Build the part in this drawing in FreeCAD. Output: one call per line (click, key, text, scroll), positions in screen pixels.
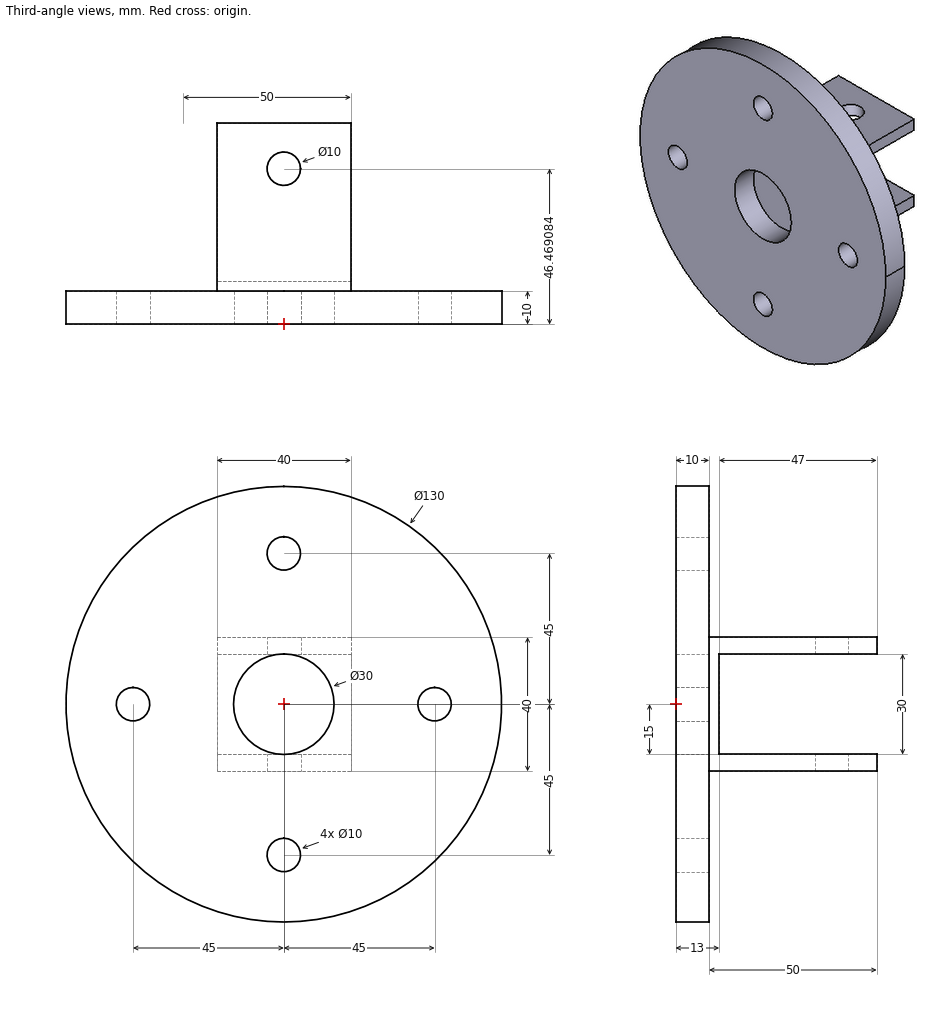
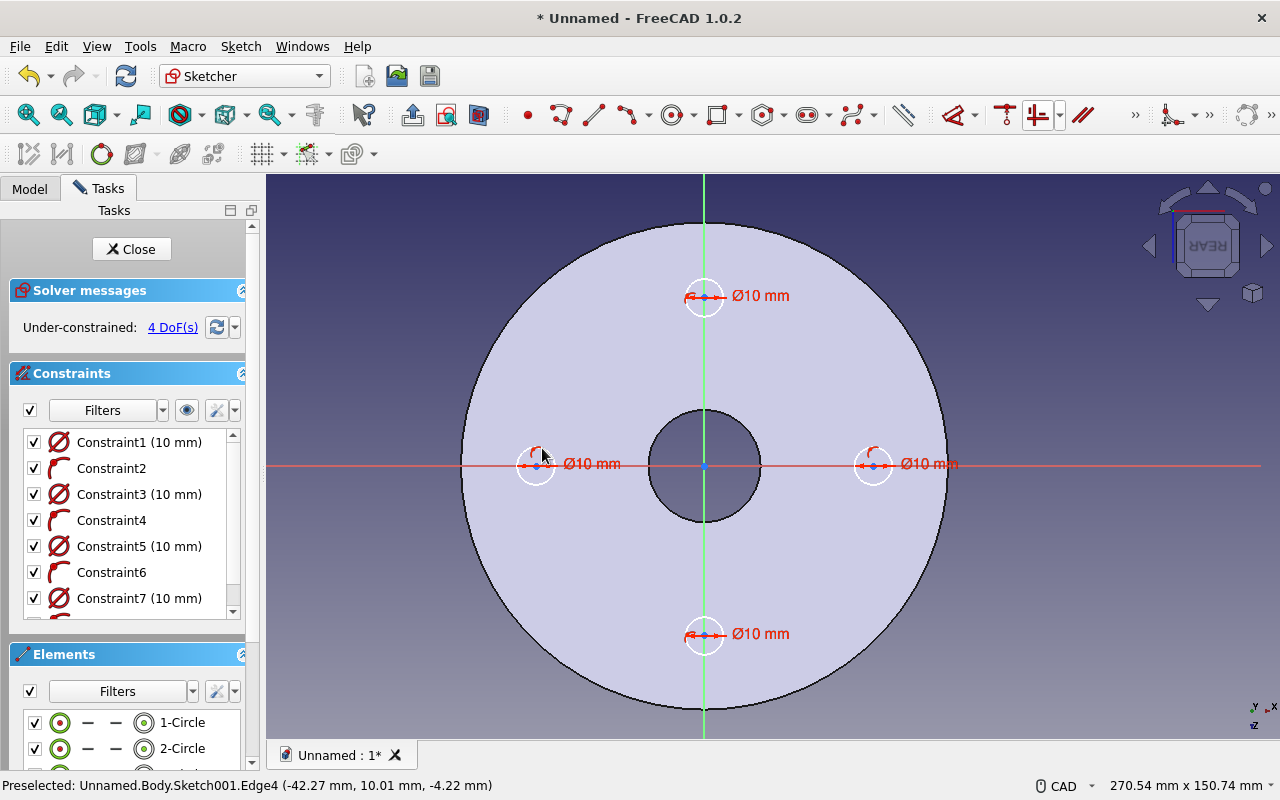
click(952, 116)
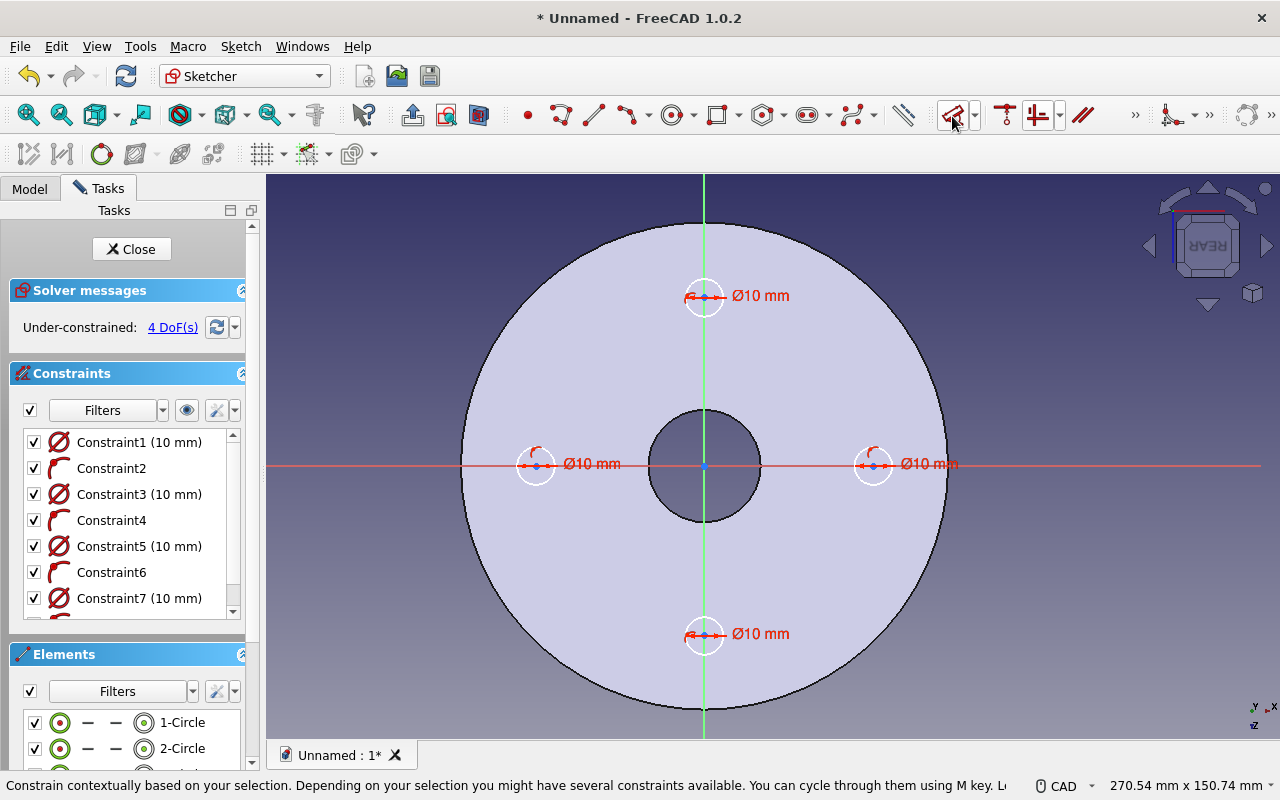
click(704, 298)
click(738, 382)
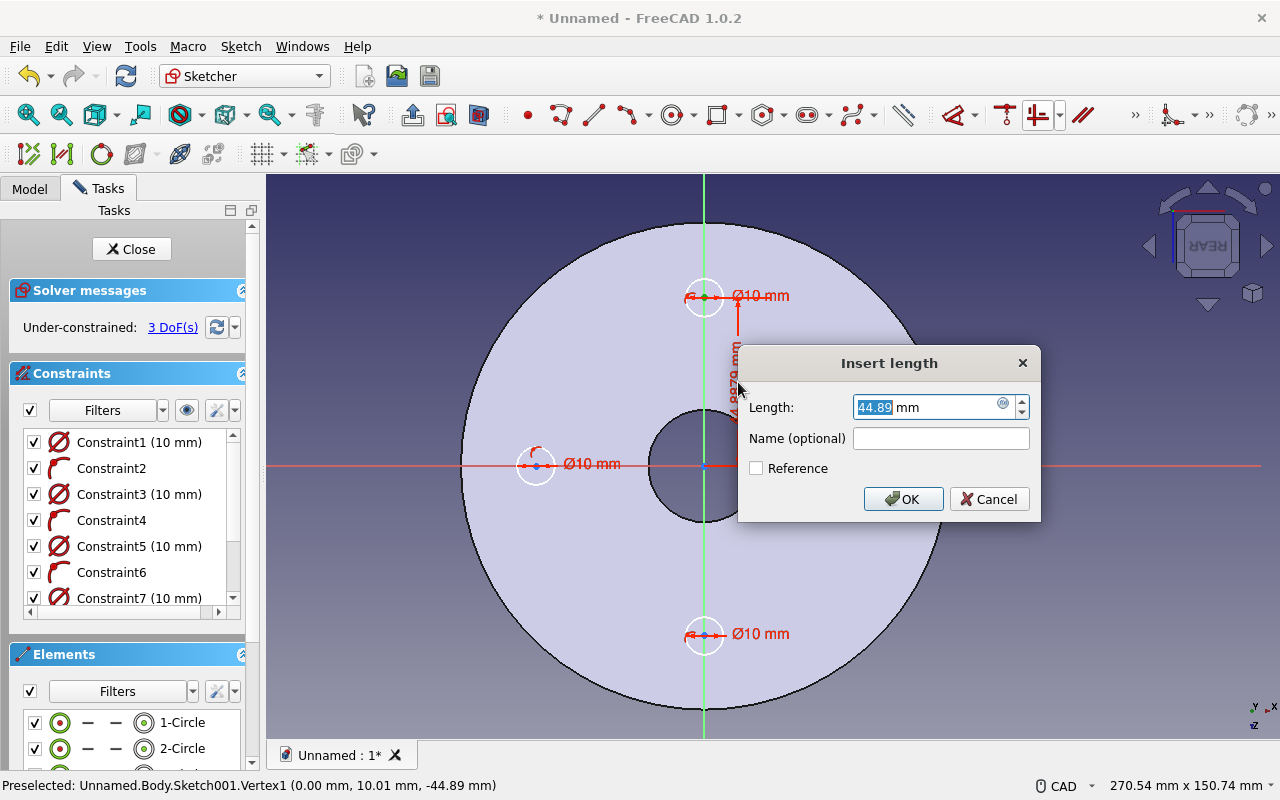
text(45)
key(Return)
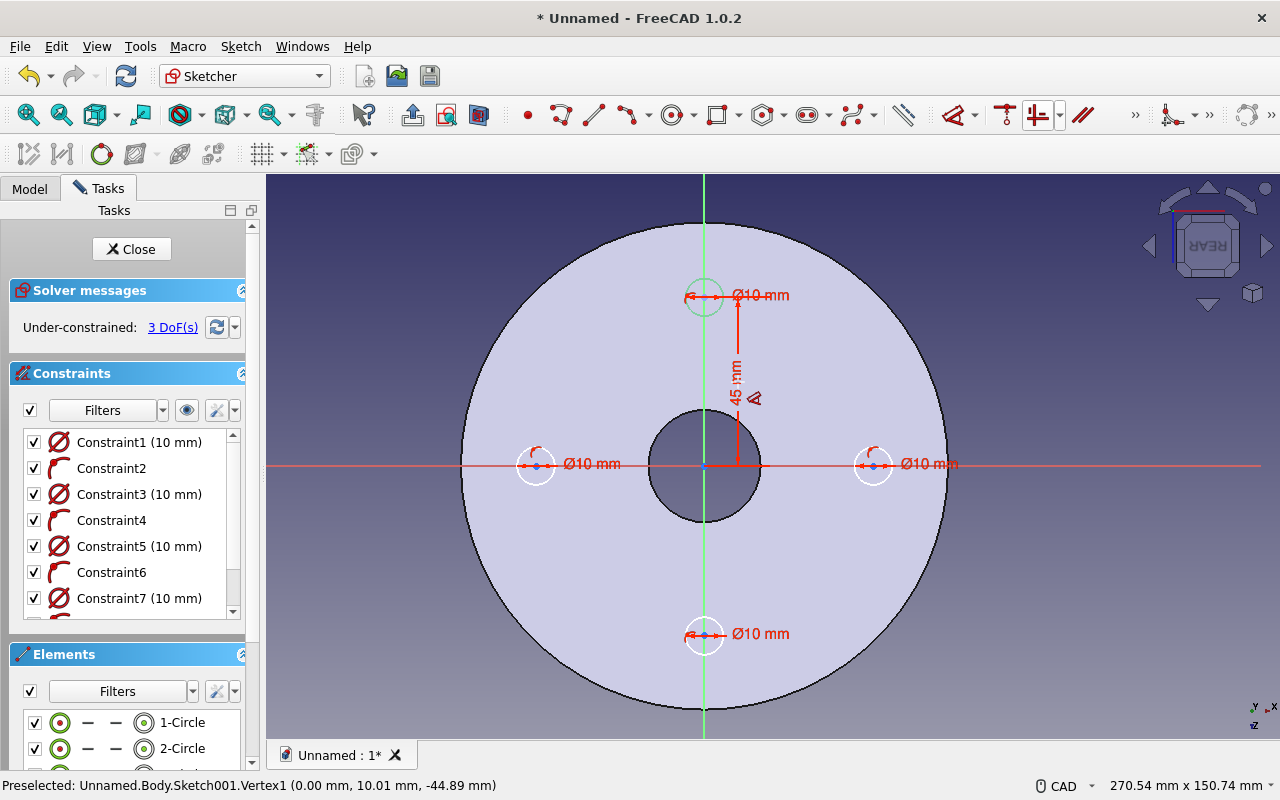
click(873, 466)
click(789, 500)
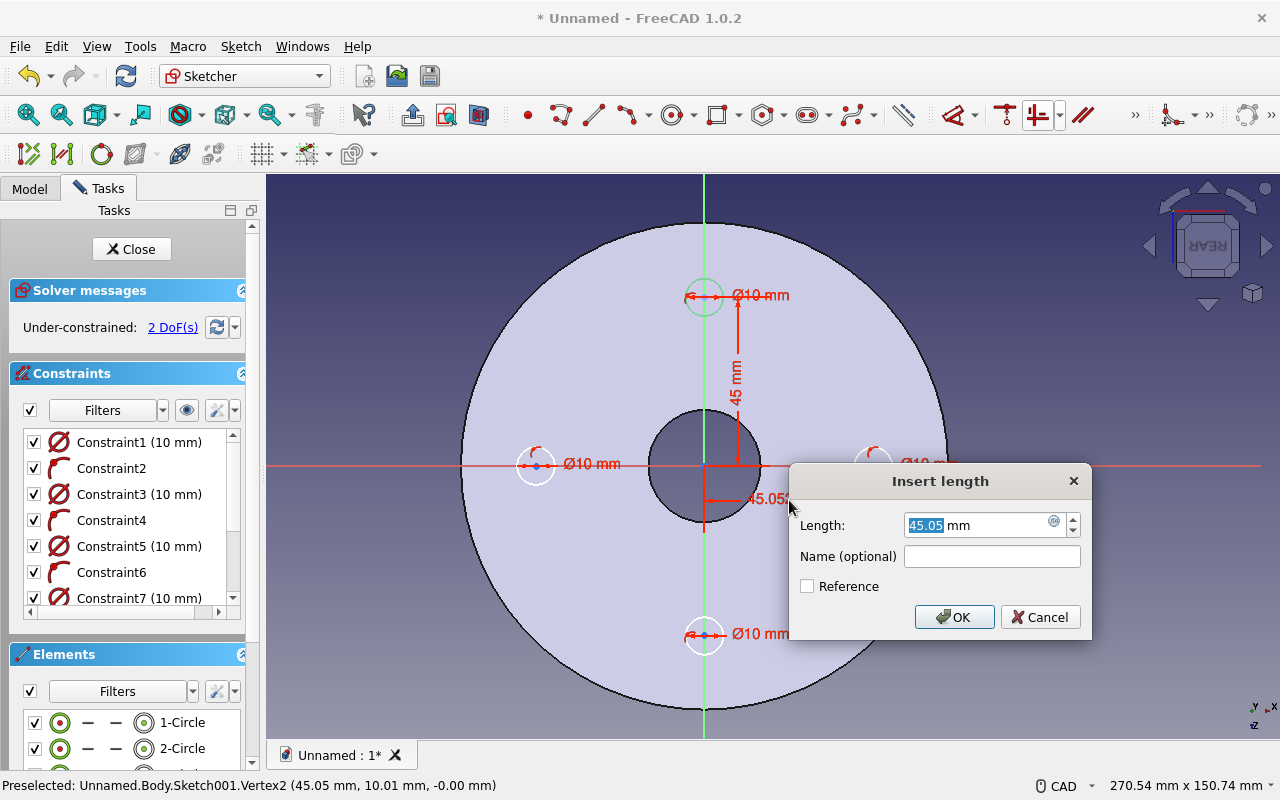
text(45)
key(Return)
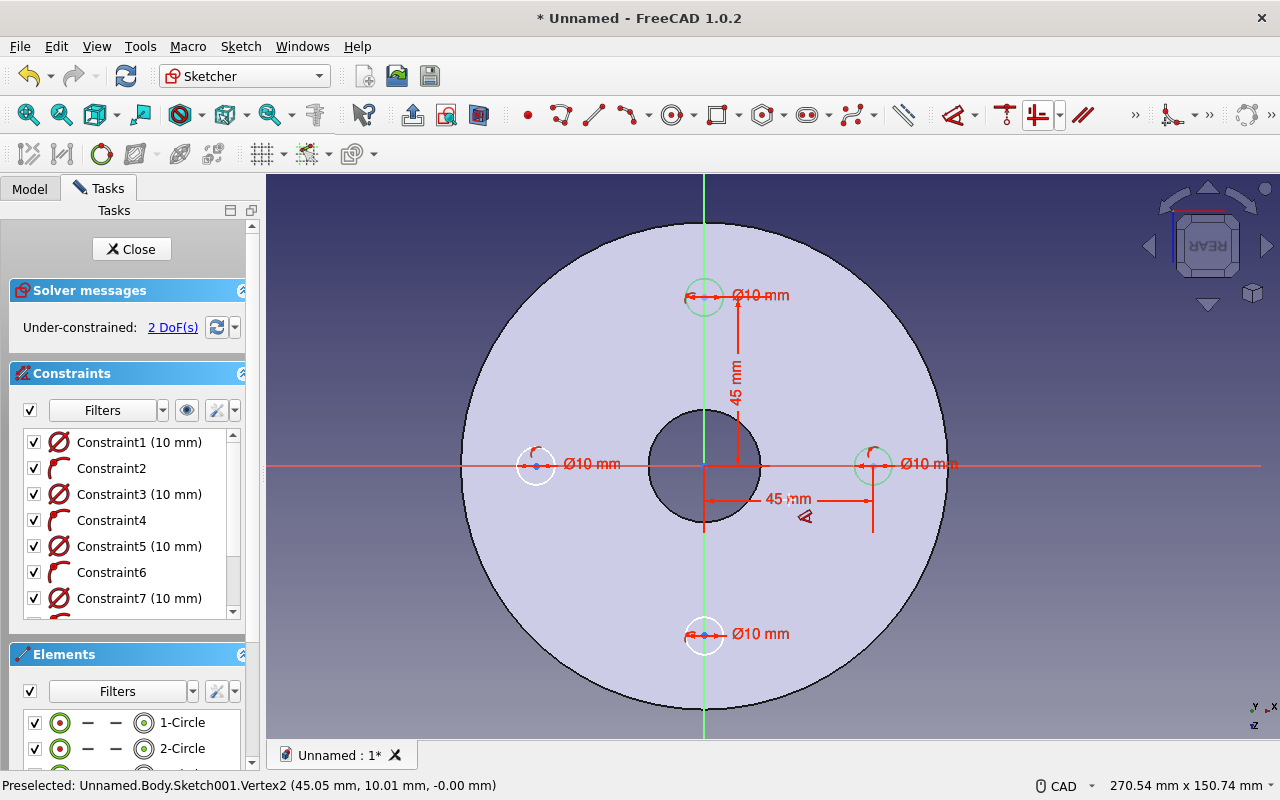
click(704, 636)
click(738, 551)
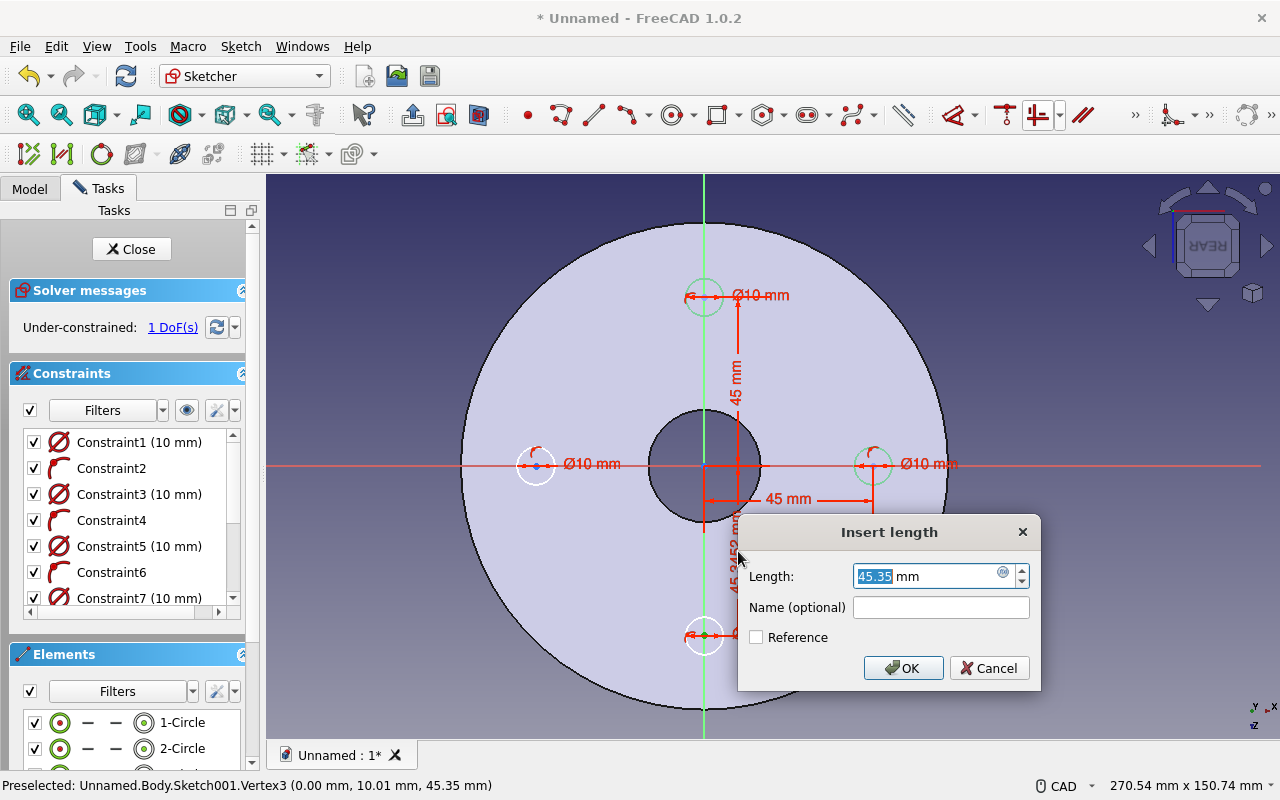
text(45)
key(Return)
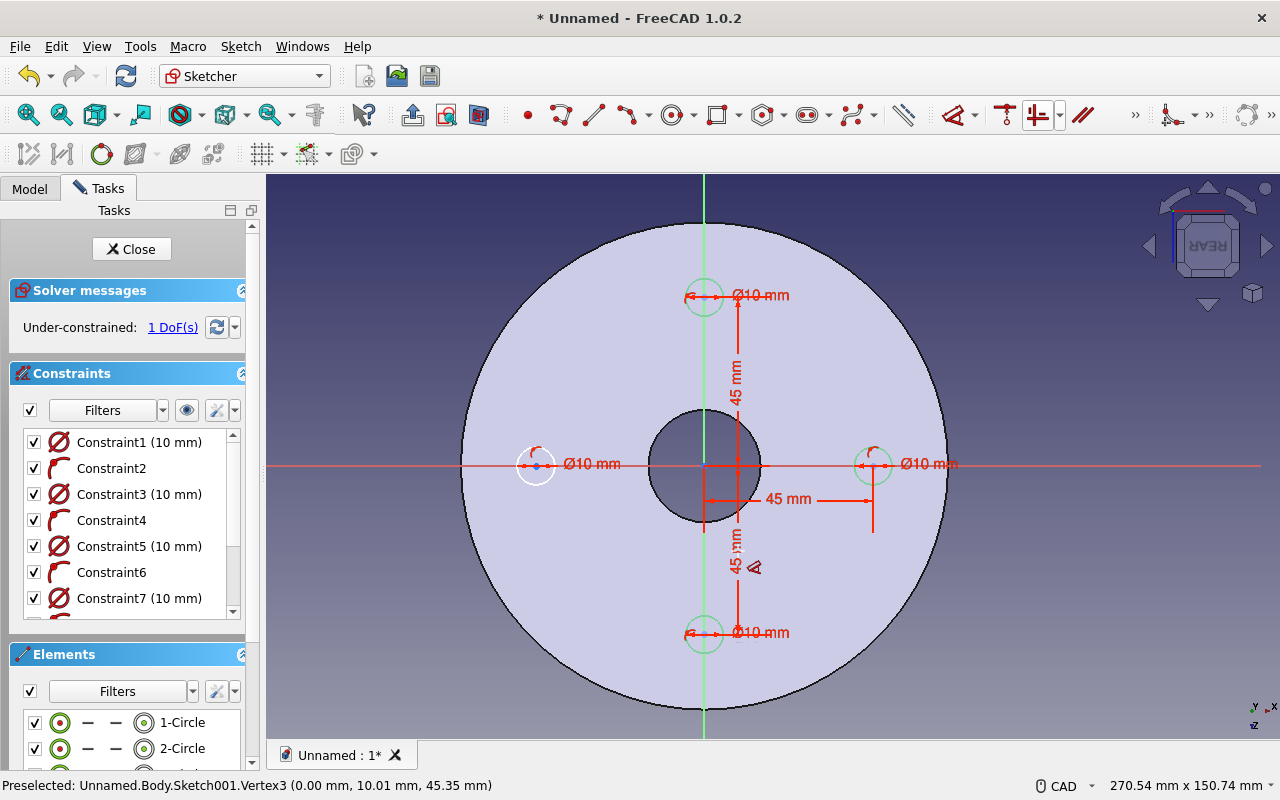
click(536, 466)
click(620, 500)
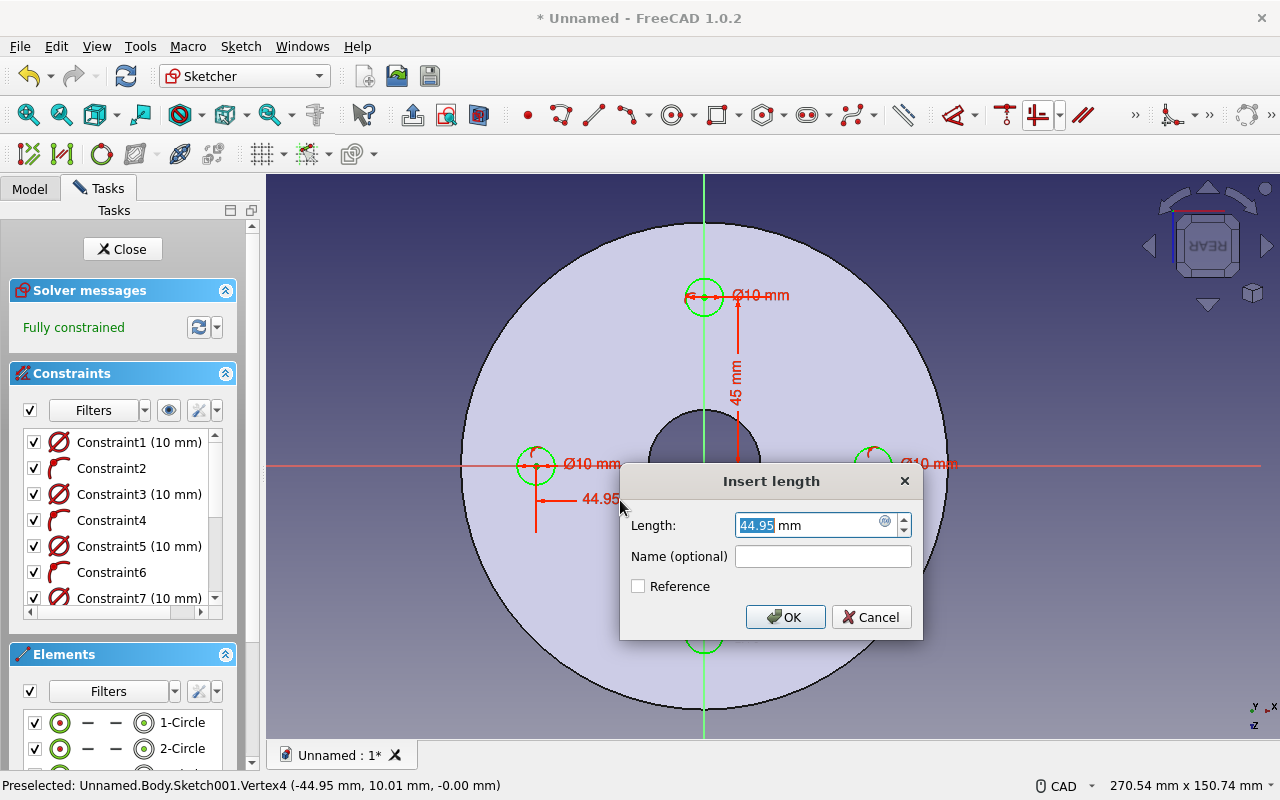
text(45)
key(Return)
key(Escape)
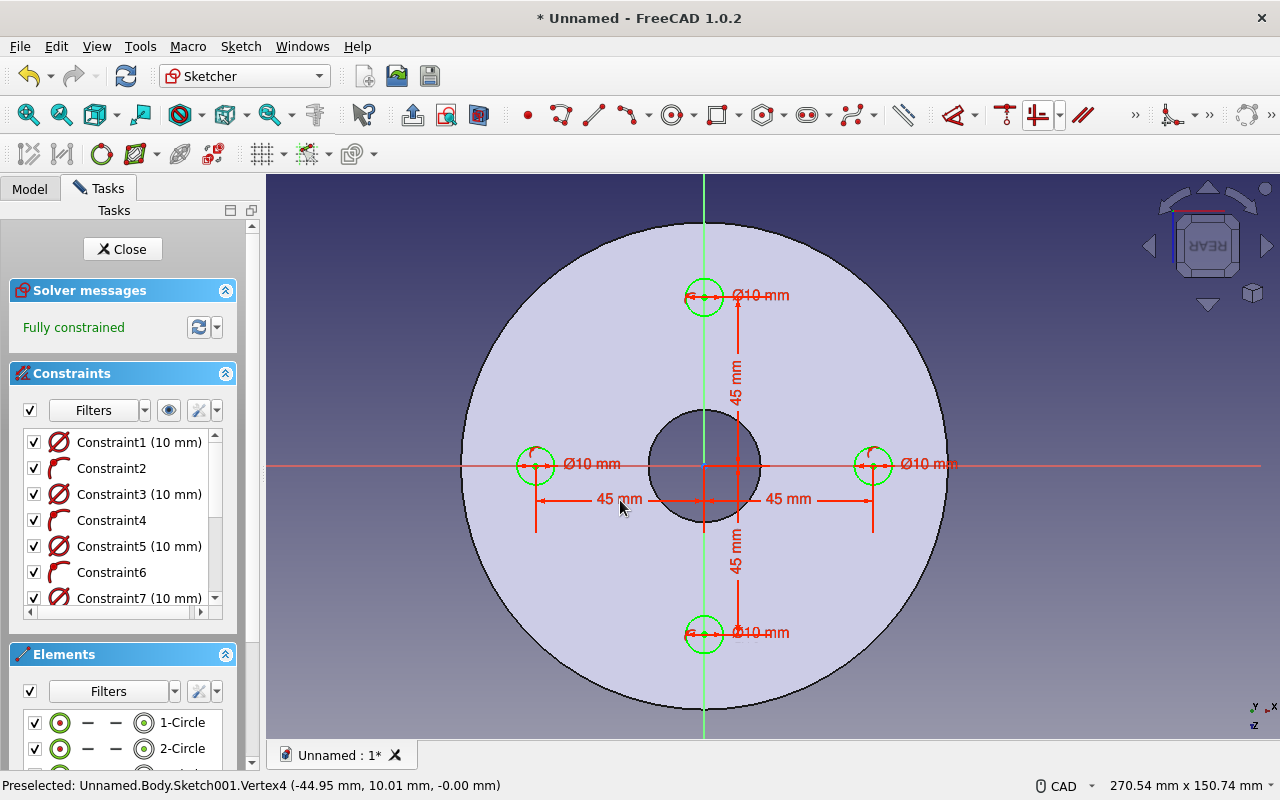
click(123, 249)